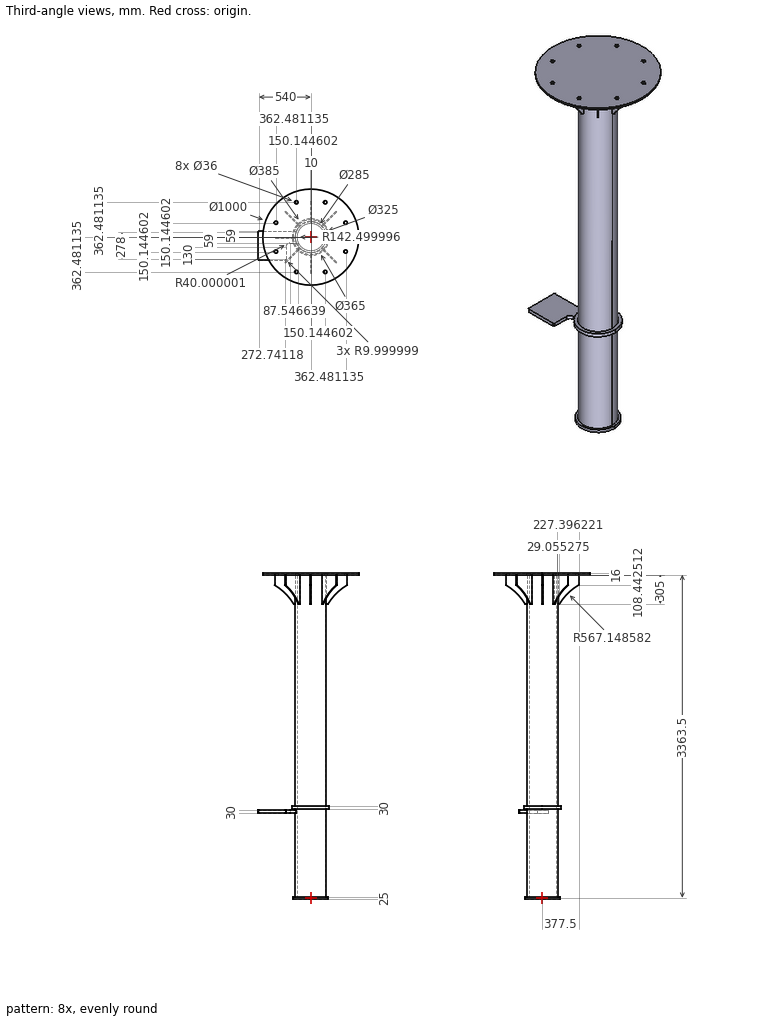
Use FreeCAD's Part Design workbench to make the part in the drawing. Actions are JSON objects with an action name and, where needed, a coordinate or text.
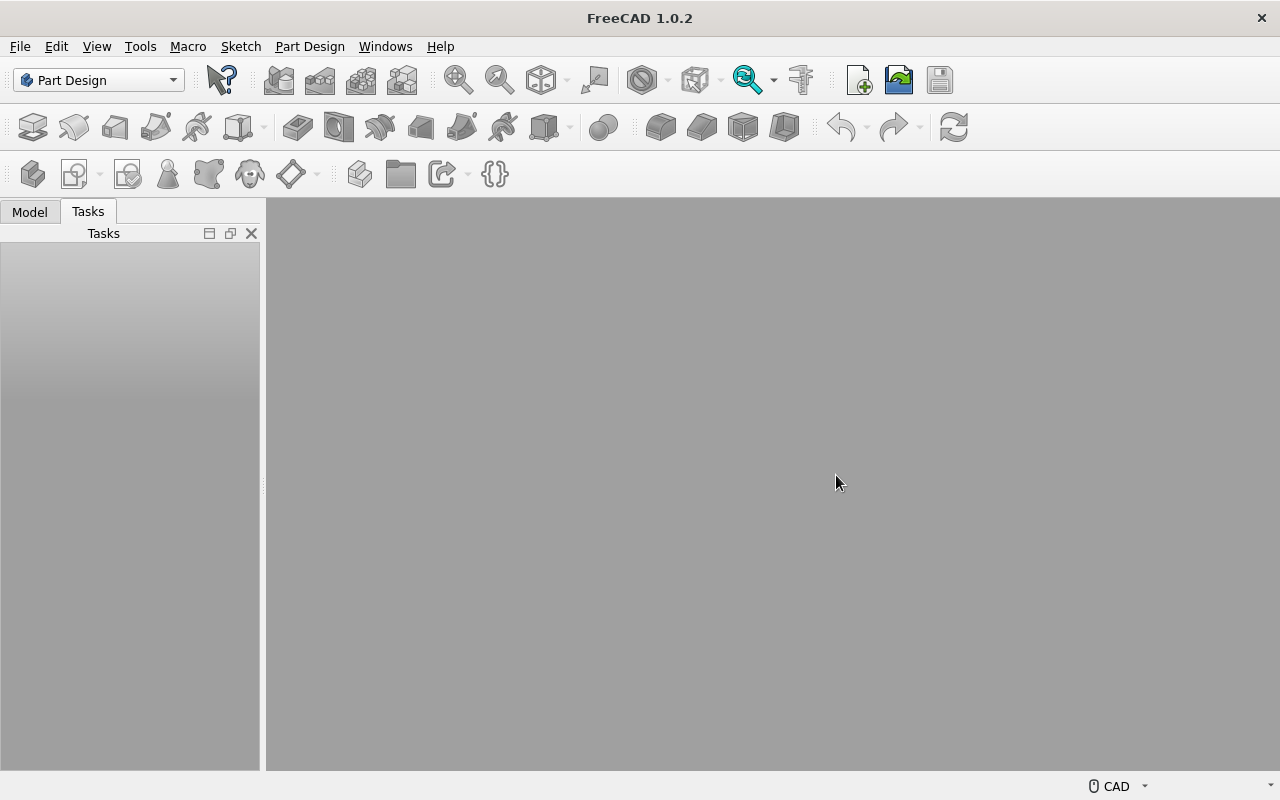
{"action": "key", "text": "ctrl+n"}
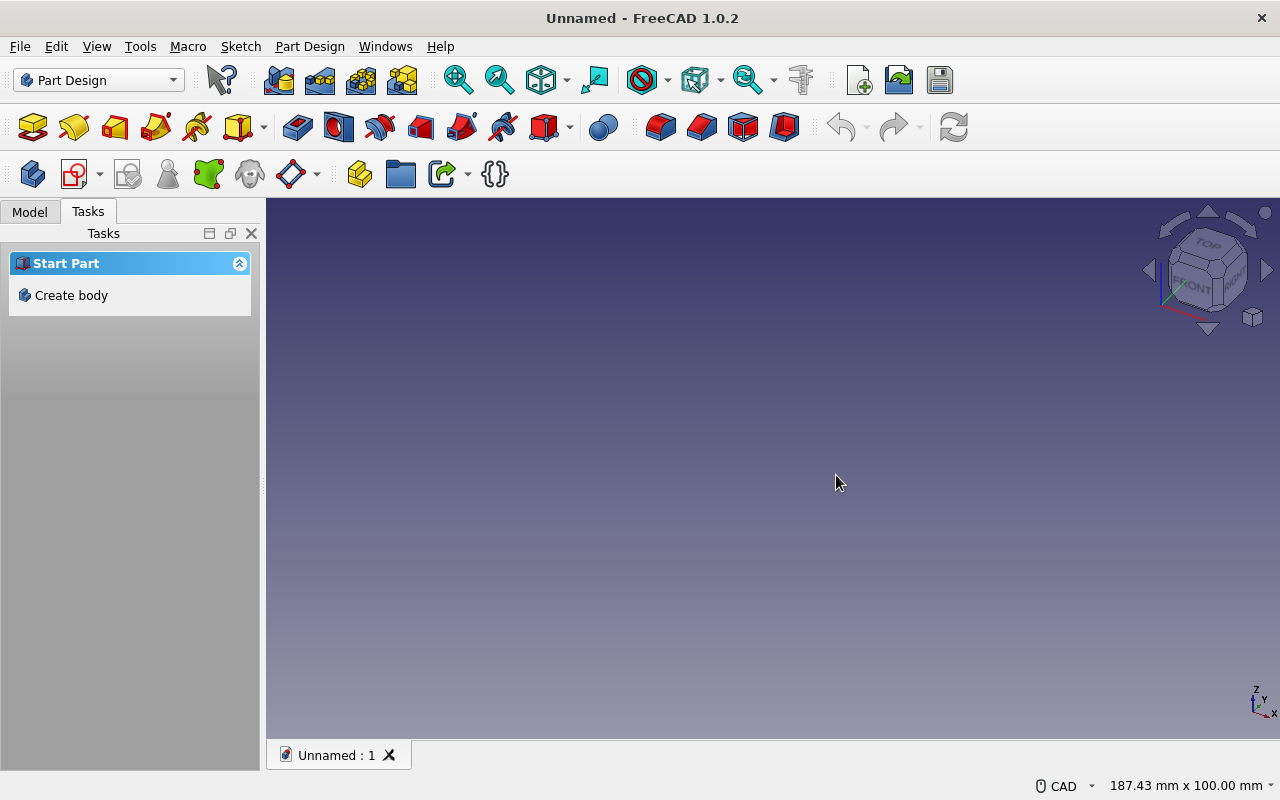
{"action": "left_click", "coordinate": [74, 174]}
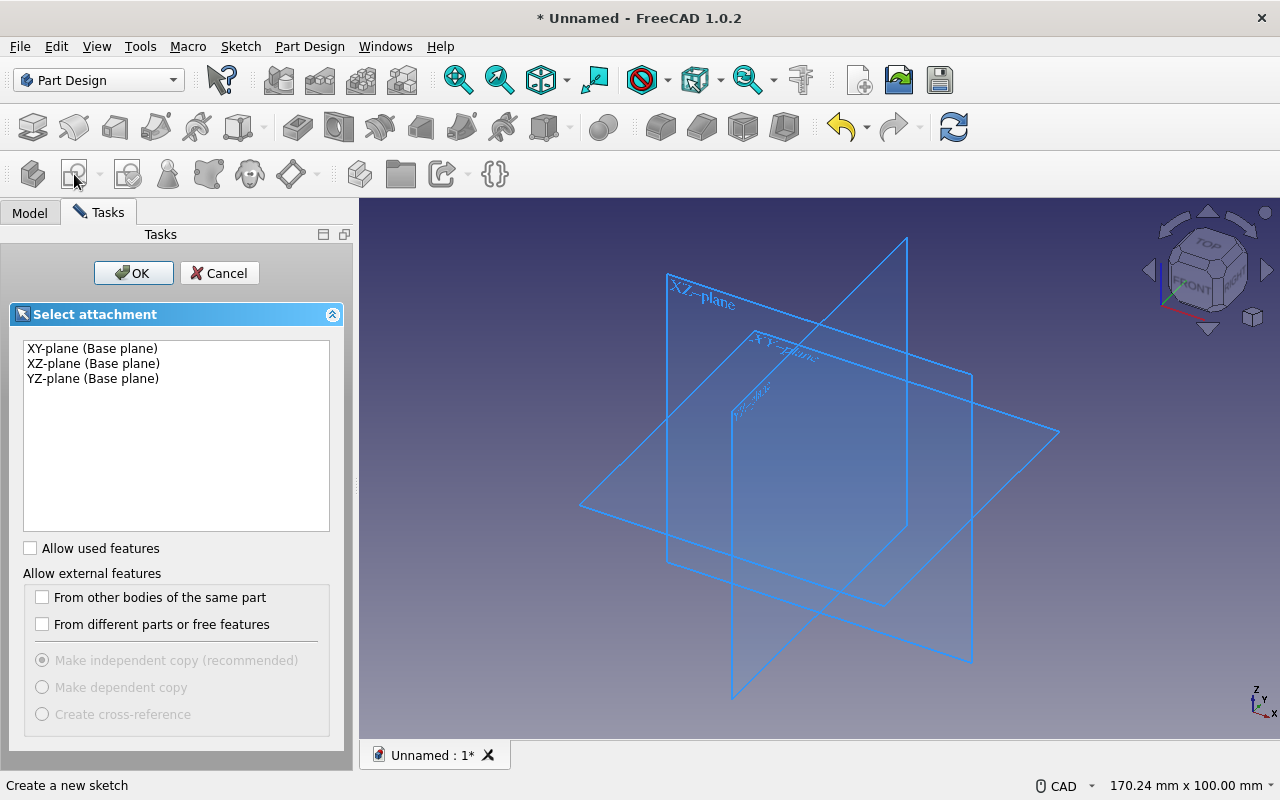
{"action": "left_click", "coordinate": [84, 348]}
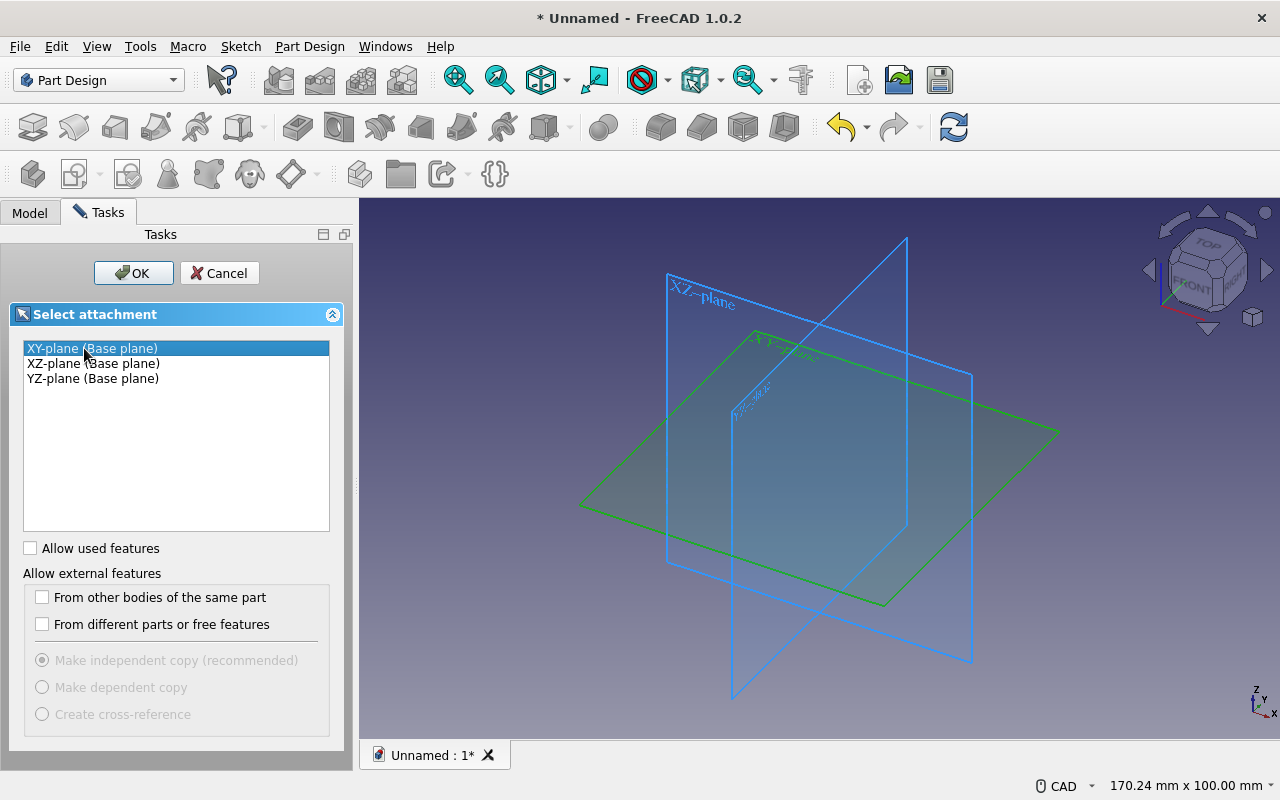
{"action": "left_click", "coordinate": [134, 273]}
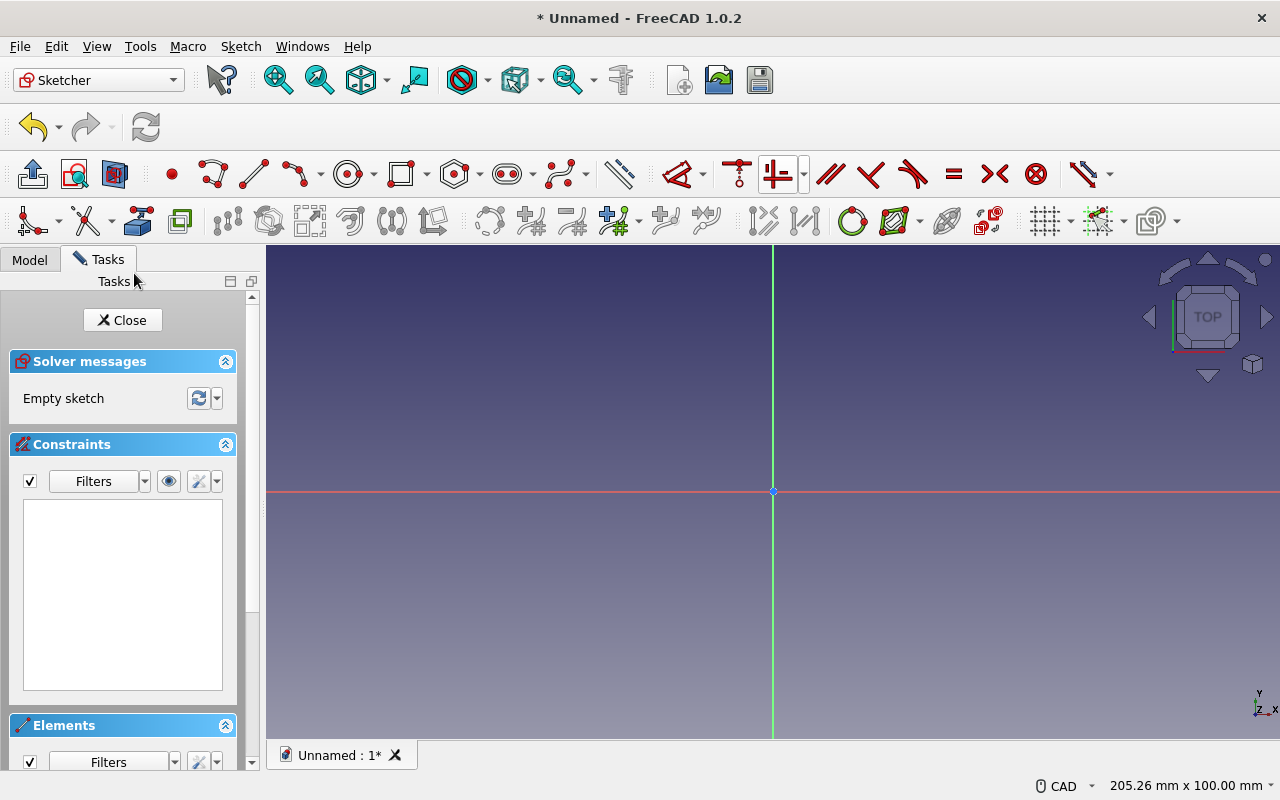
{"action": "scroll", "coordinate": [687, 492], "scroll_direction": "down", "scroll_amount": 8}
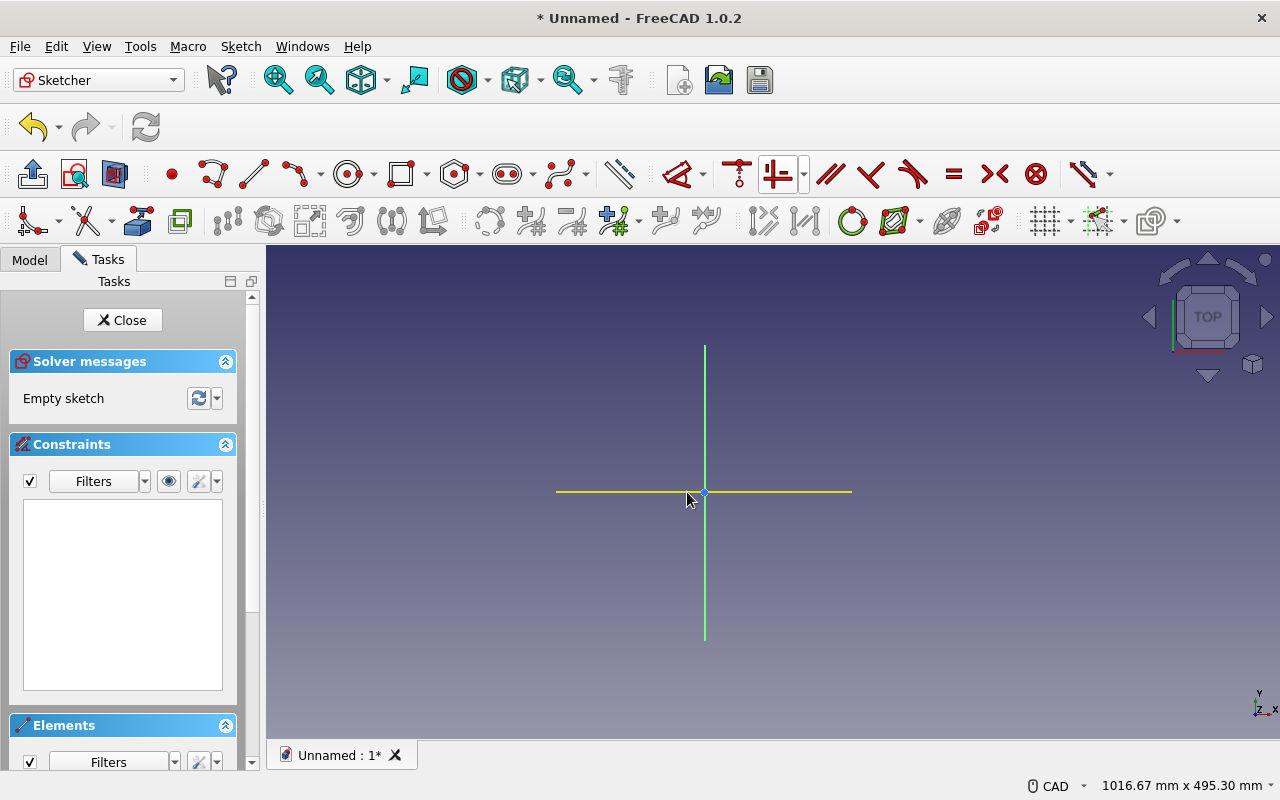
{"action": "key", "text": "g c"}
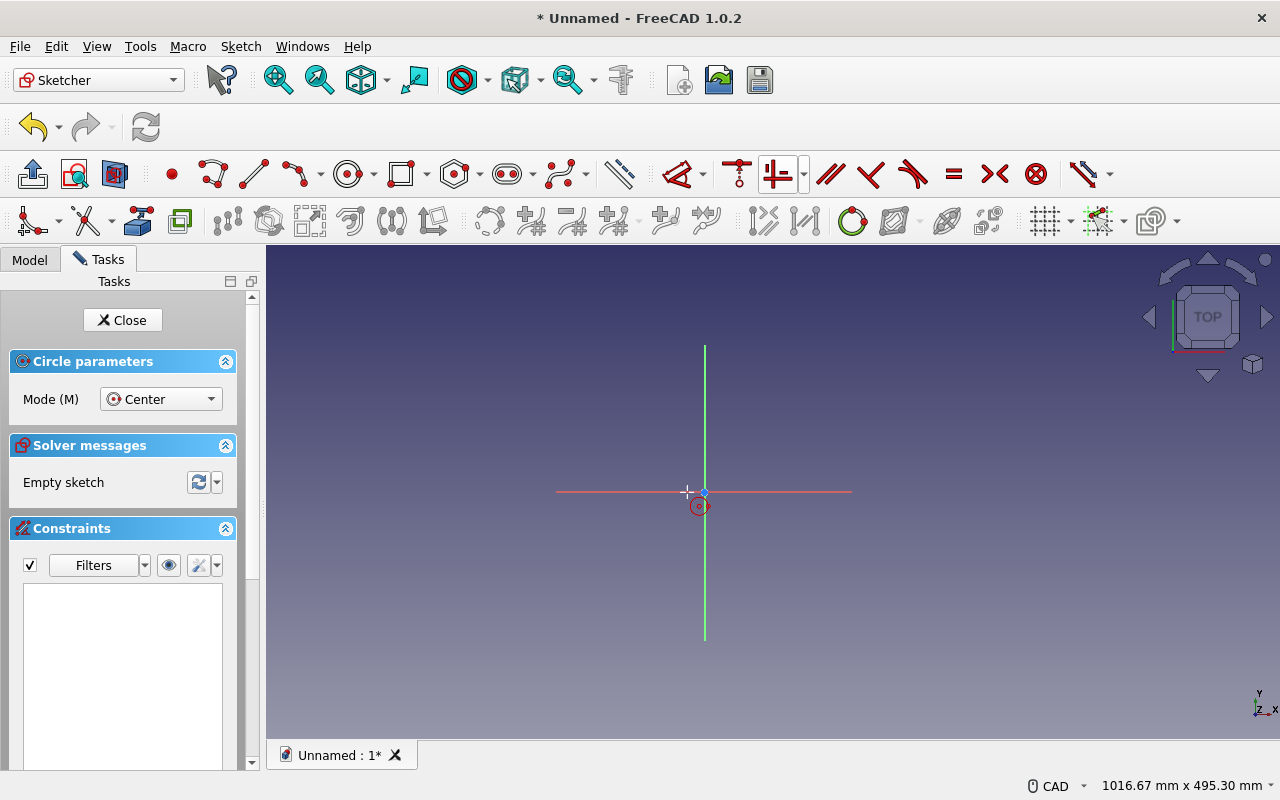
{"action": "left_click", "coordinate": [705, 492]}
{"action": "left_click", "coordinate": [819, 378]}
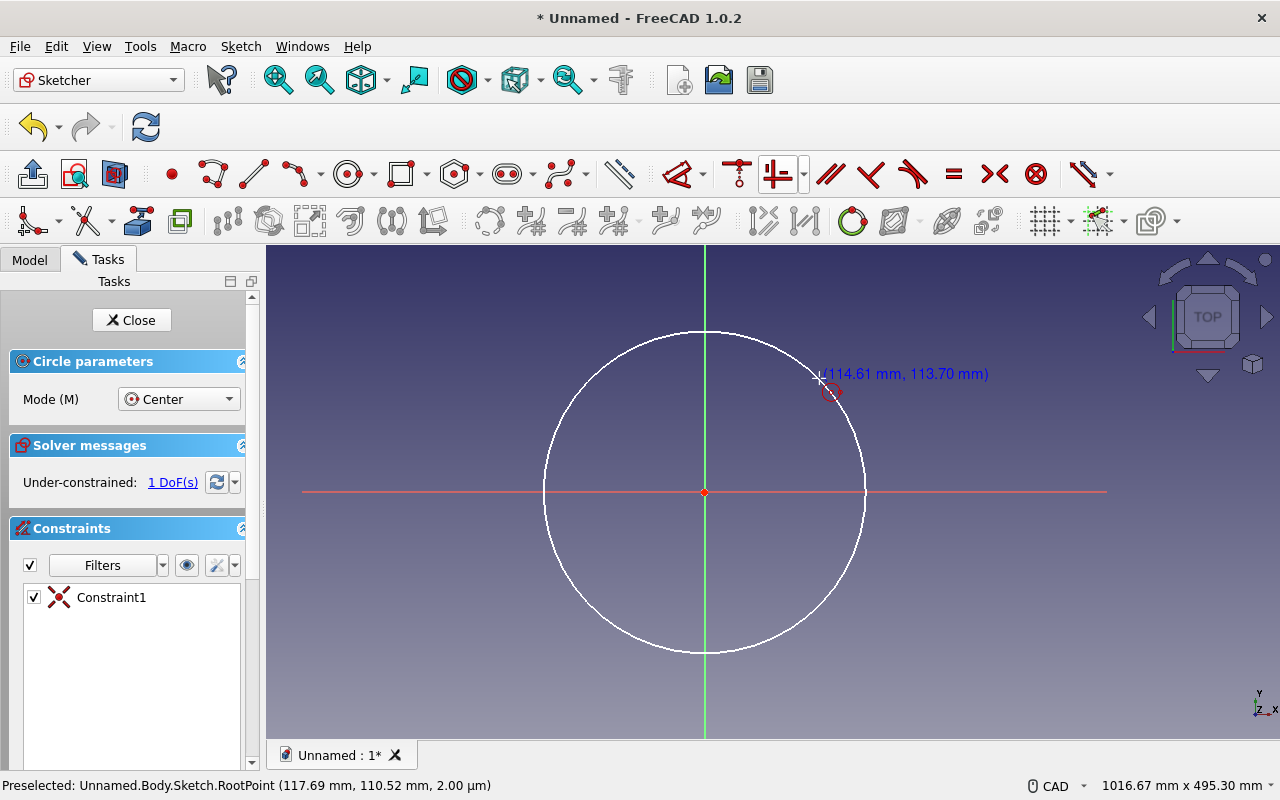
{"action": "left_click", "coordinate": [705, 492]}
{"action": "left_click", "coordinate": [805, 392]}
{"action": "key", "text": "Escape"}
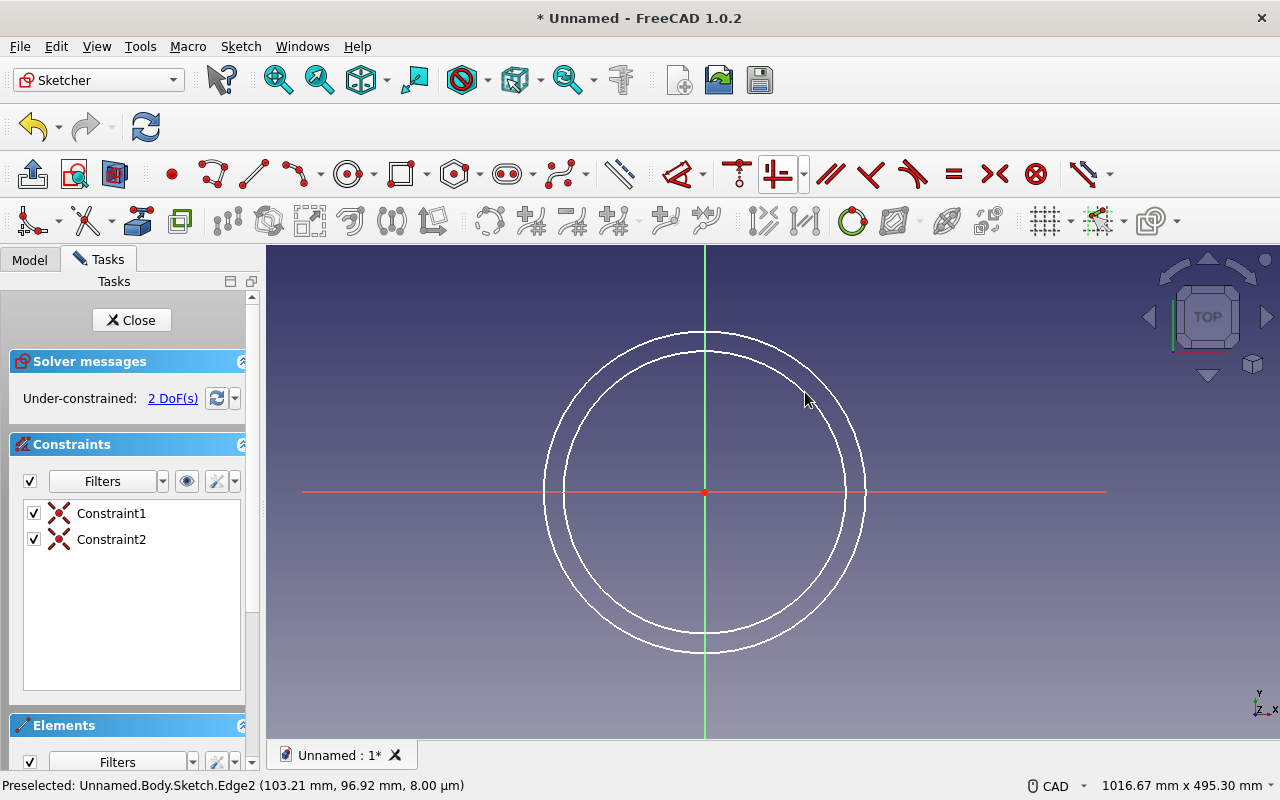
{"action": "left_click", "coordinate": [818, 378]}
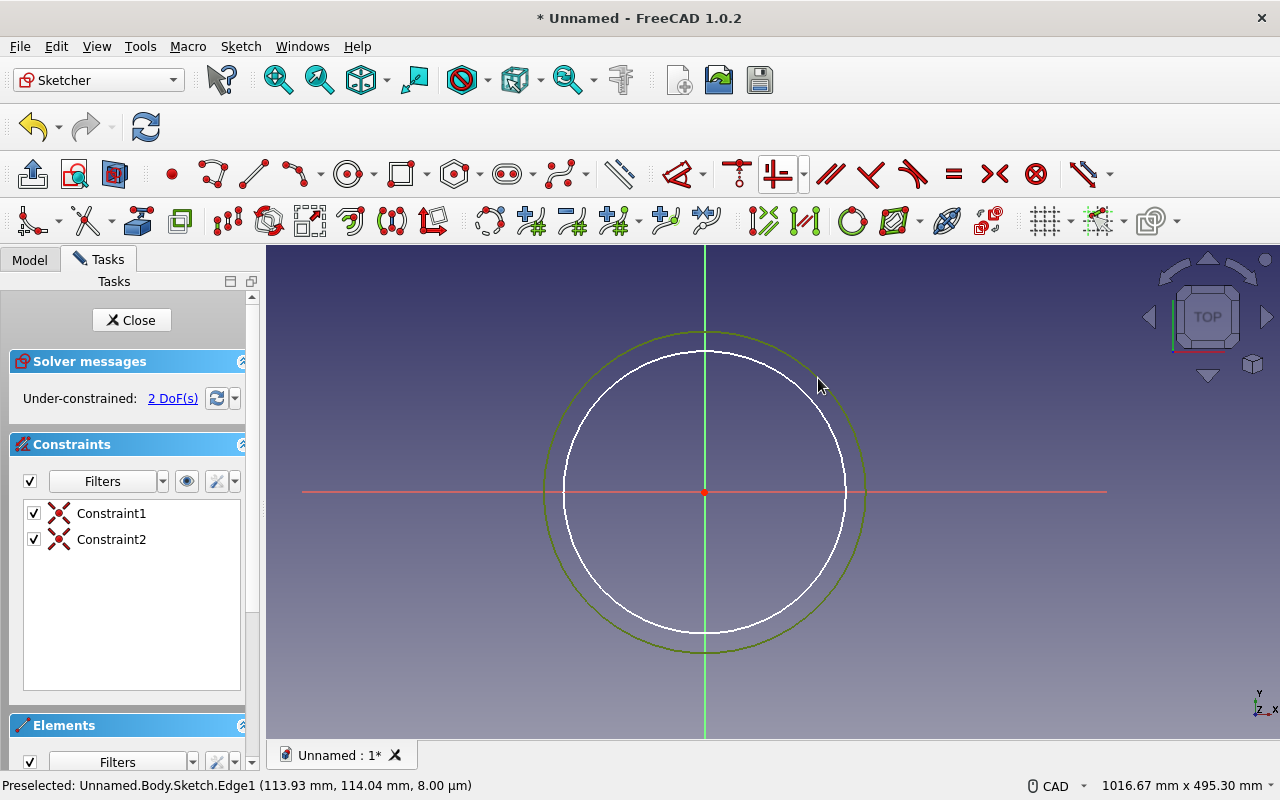
{"action": "key", "text": "k o"}